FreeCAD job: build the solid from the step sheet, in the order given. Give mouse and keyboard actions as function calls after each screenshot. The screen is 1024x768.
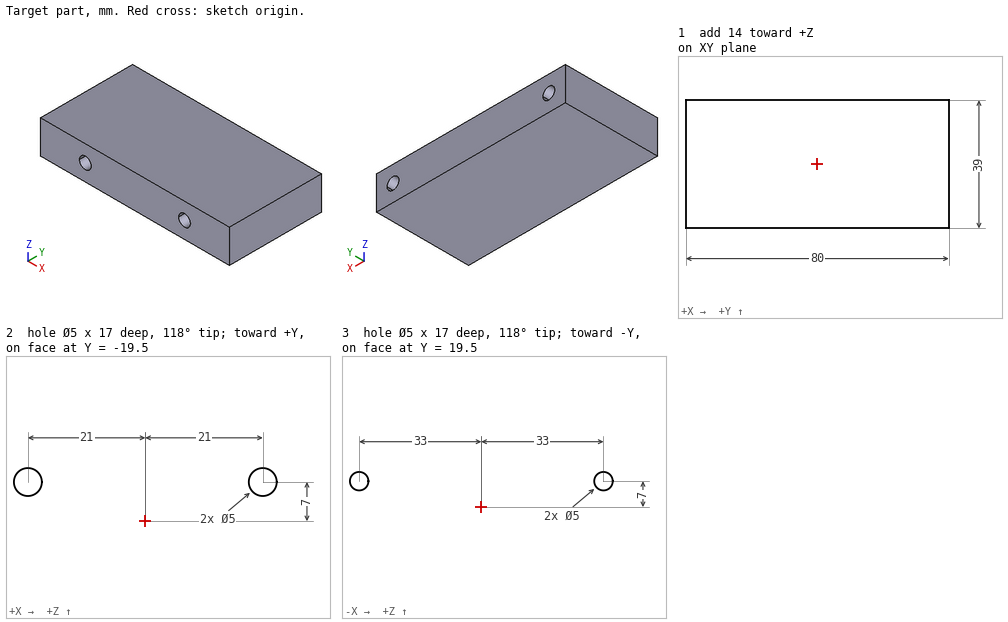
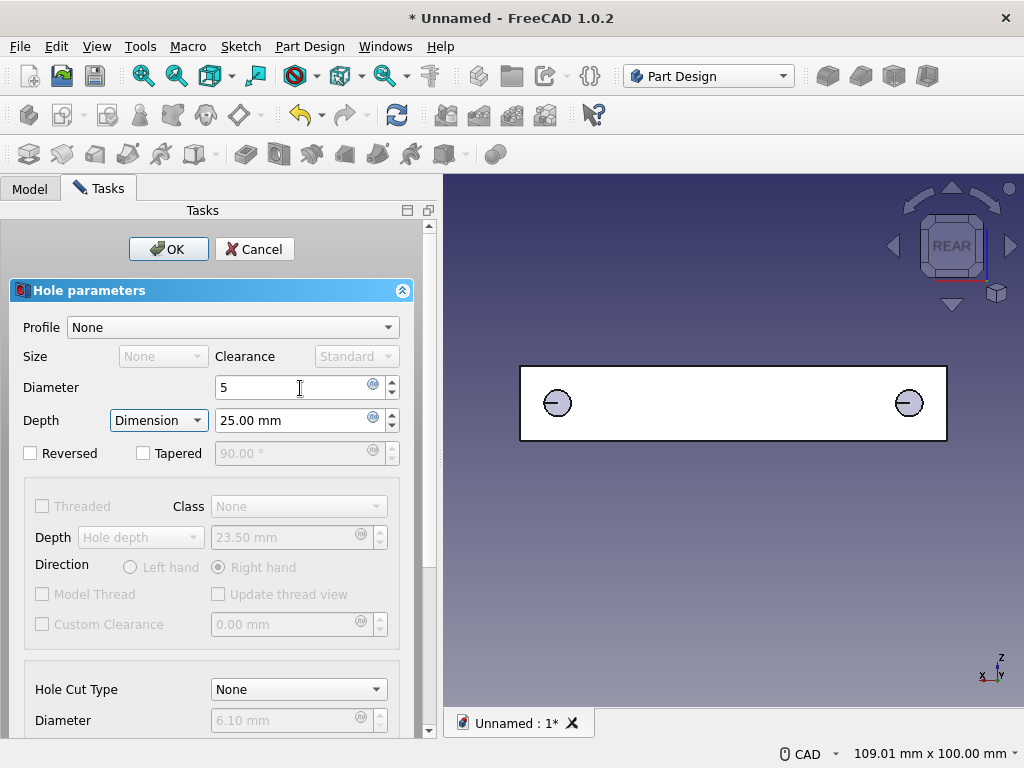
triple_click(300, 420)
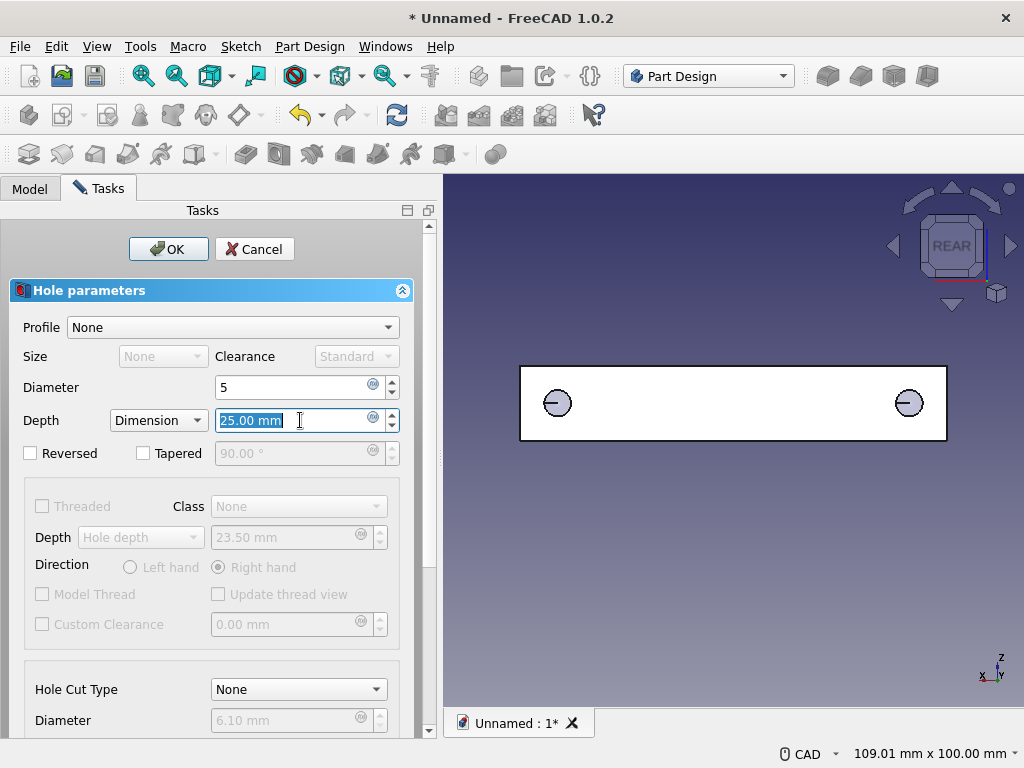
text(17)
key(Tab)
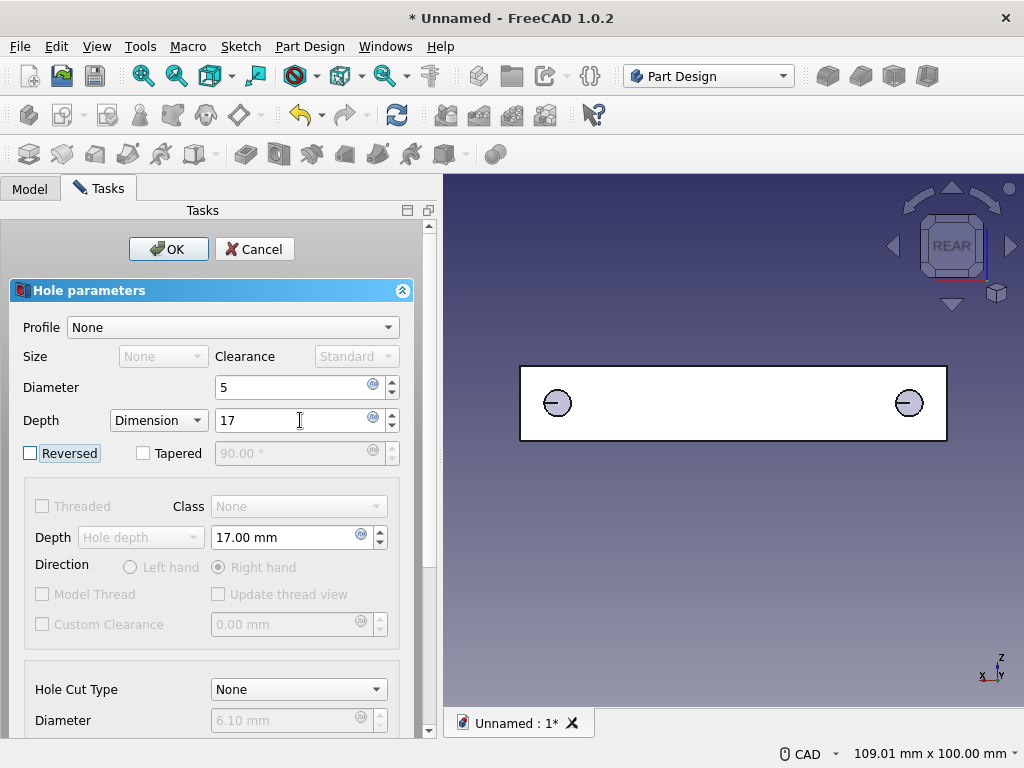
click(169, 249)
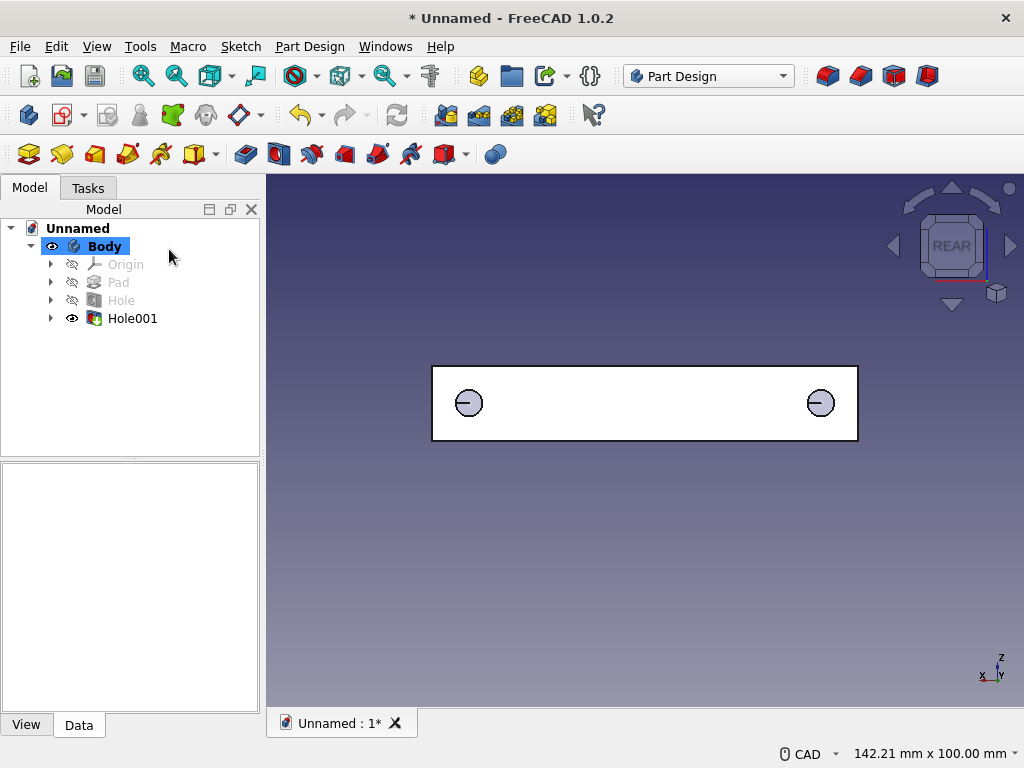
key(0)